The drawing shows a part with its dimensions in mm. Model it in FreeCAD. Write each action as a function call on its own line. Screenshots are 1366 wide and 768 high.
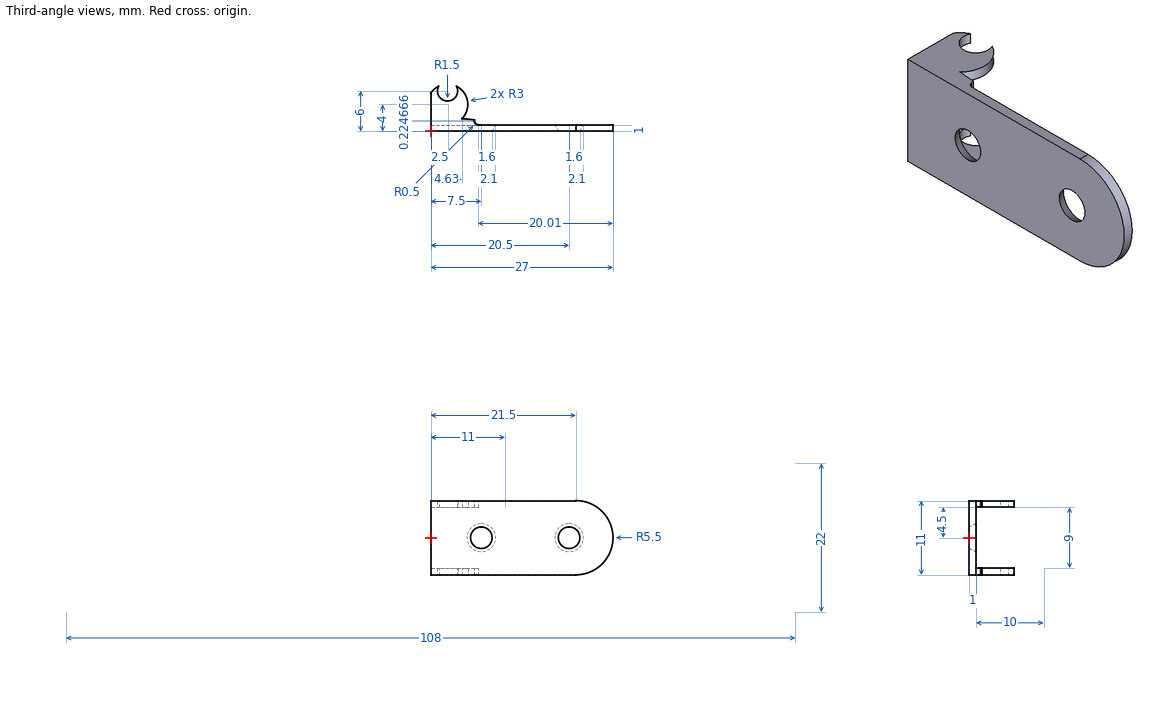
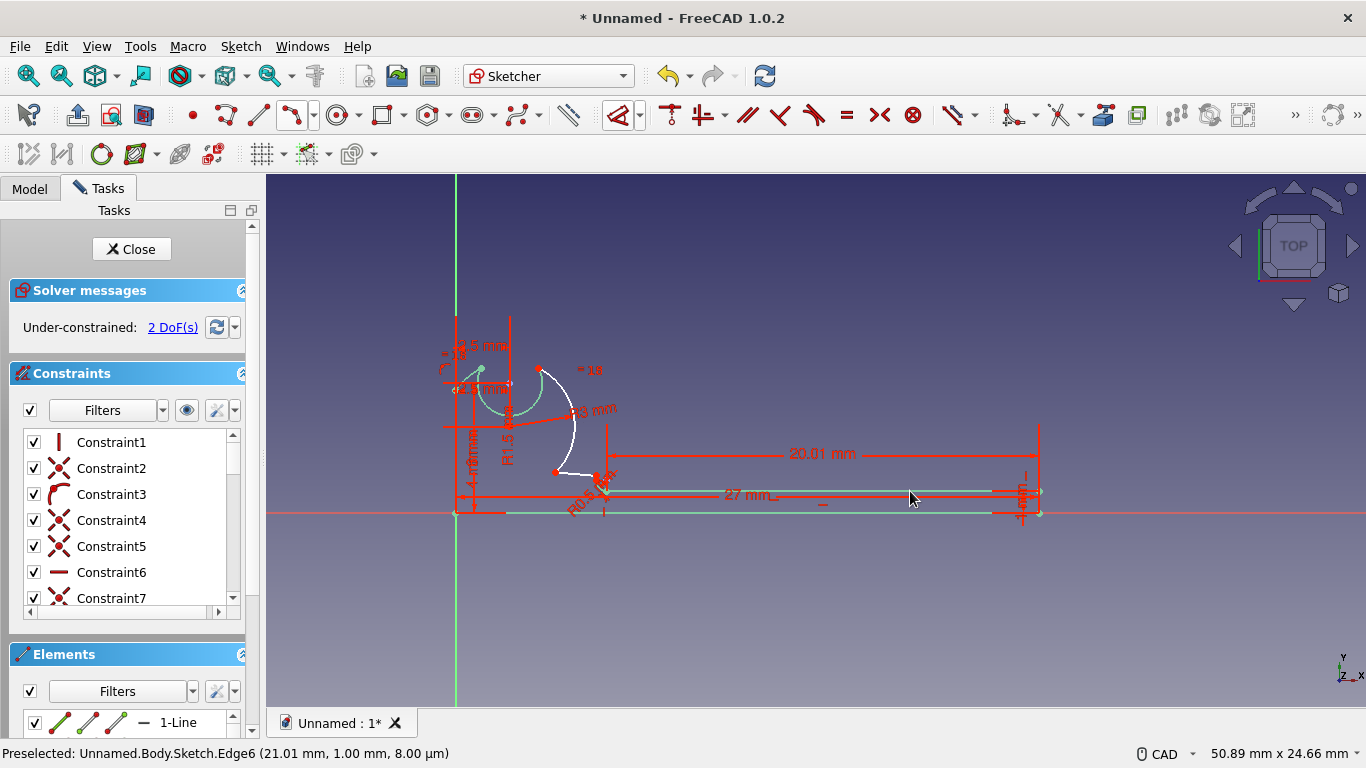
click(556, 472)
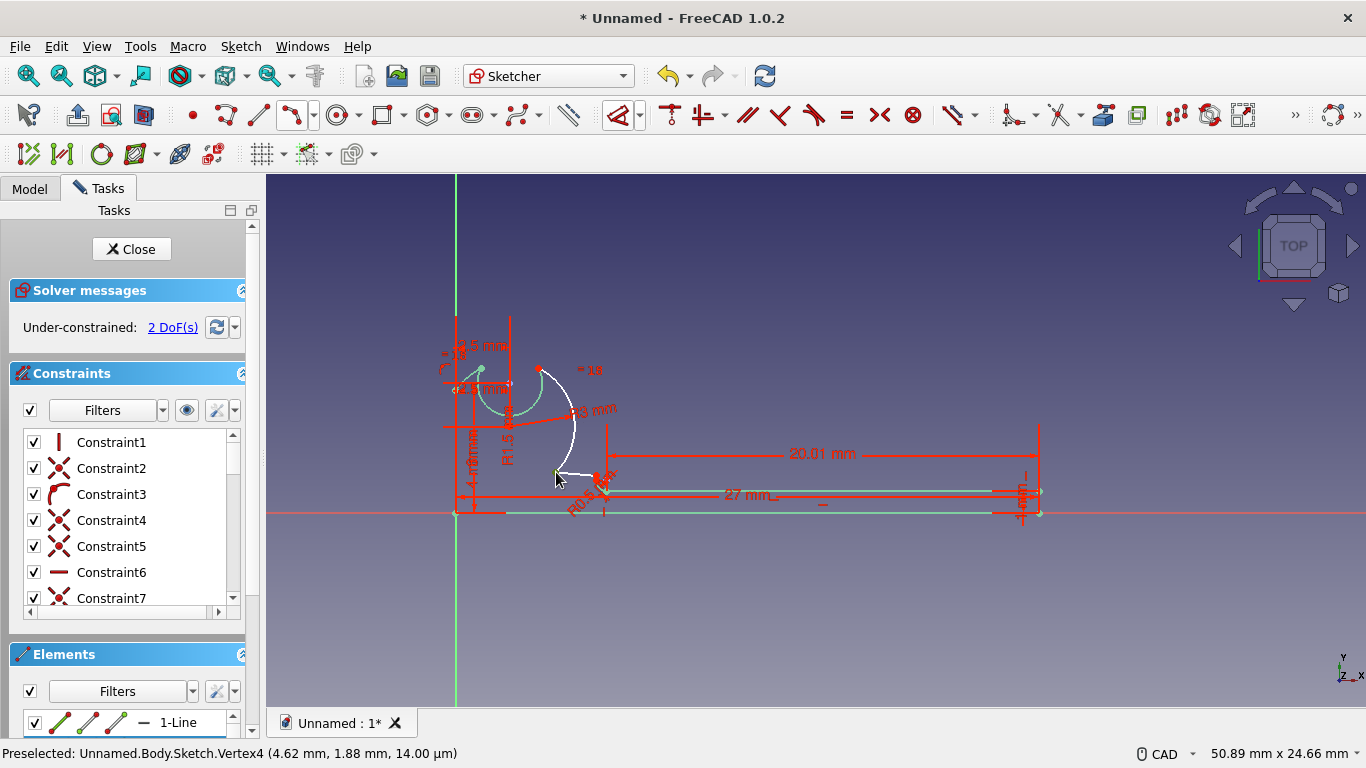
key(l)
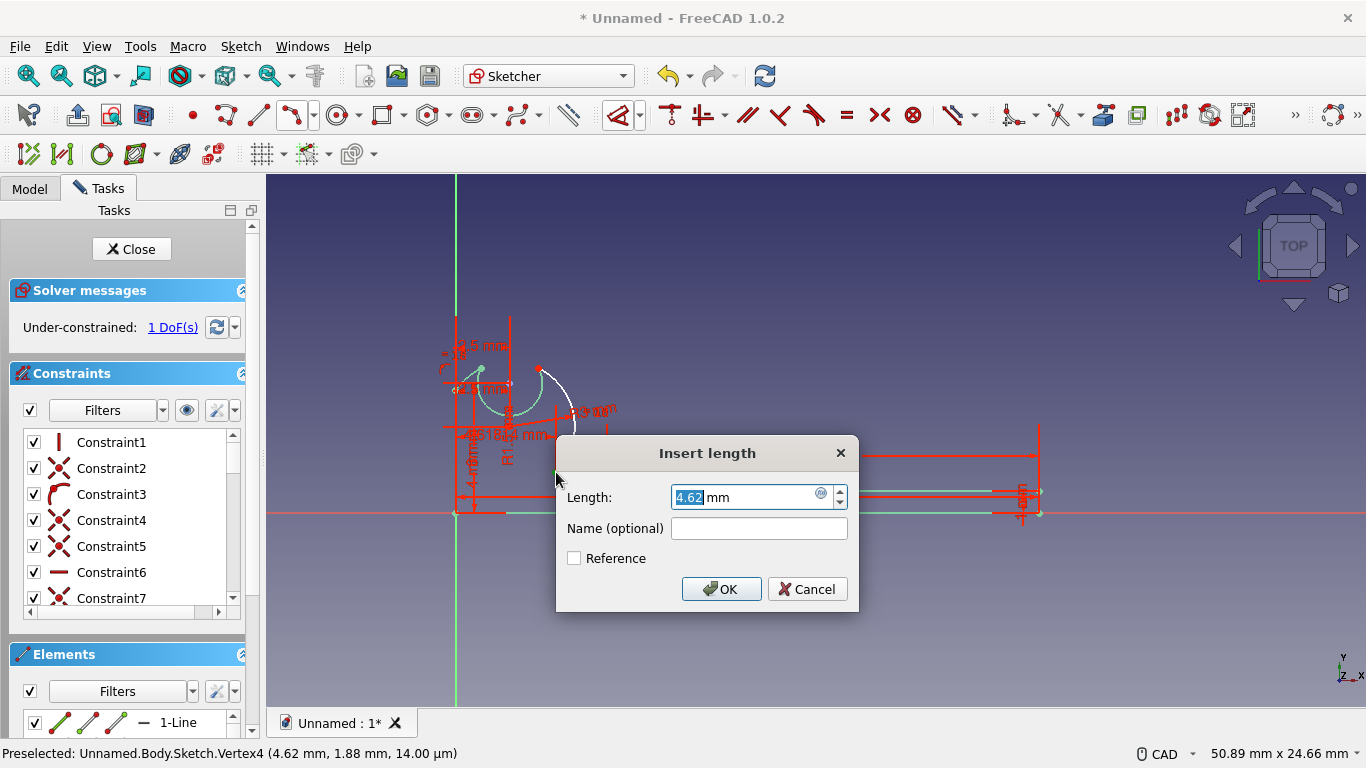
text(4.63)
key(Return)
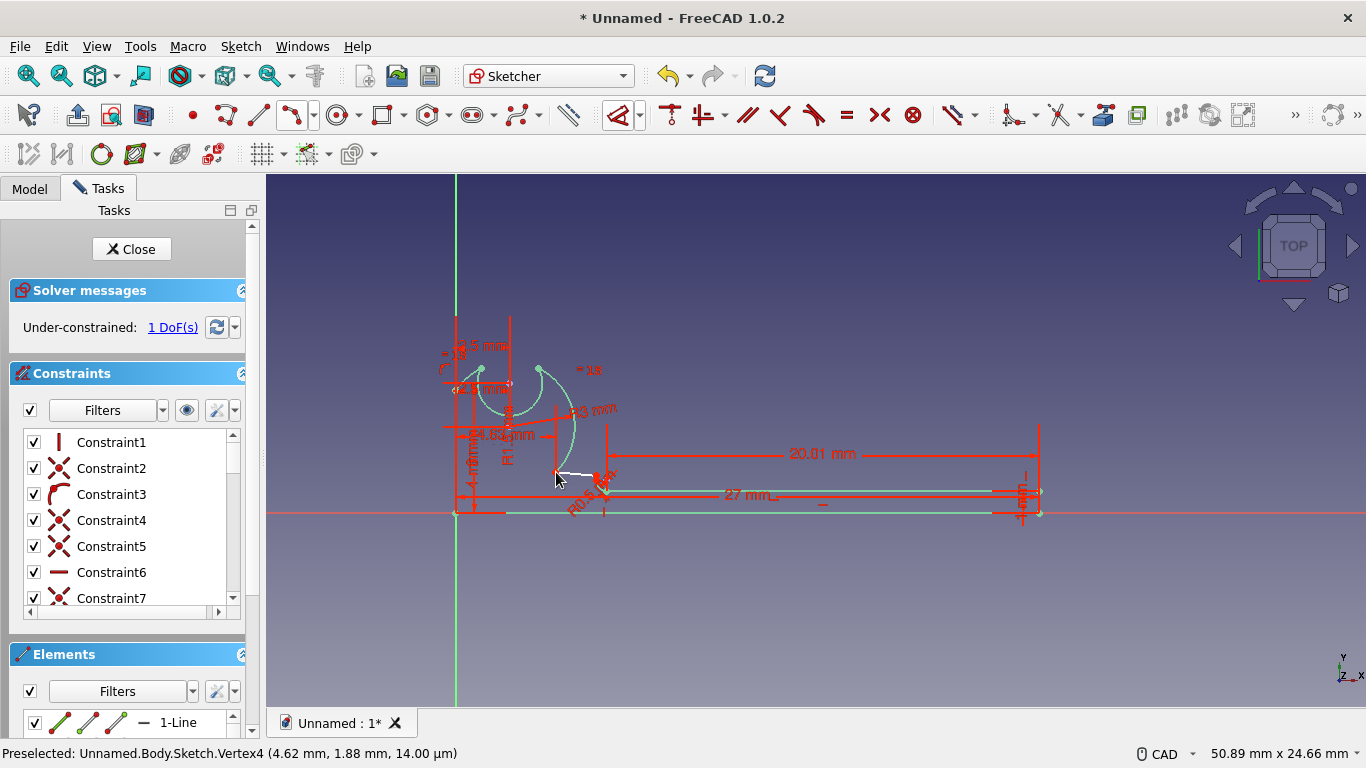
scroll(596, 478, up, 11)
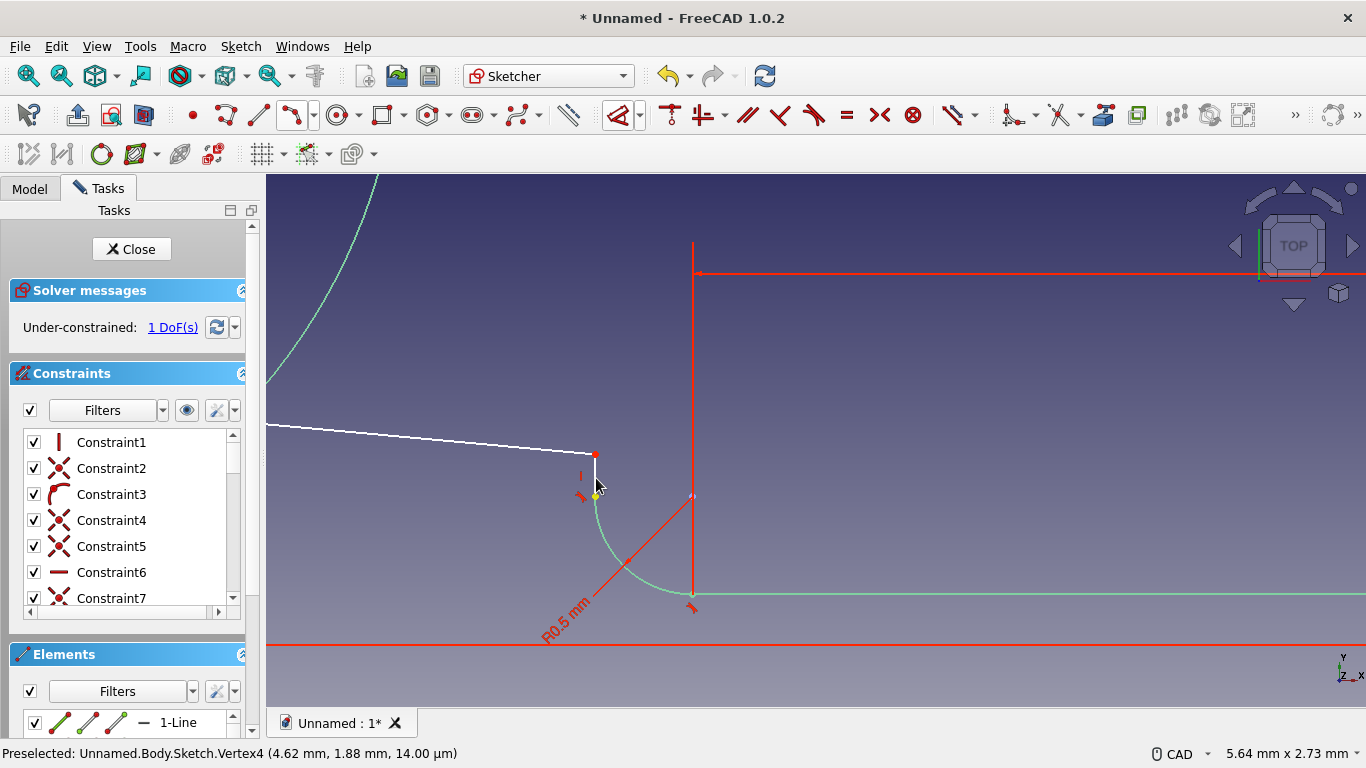
click(595, 476)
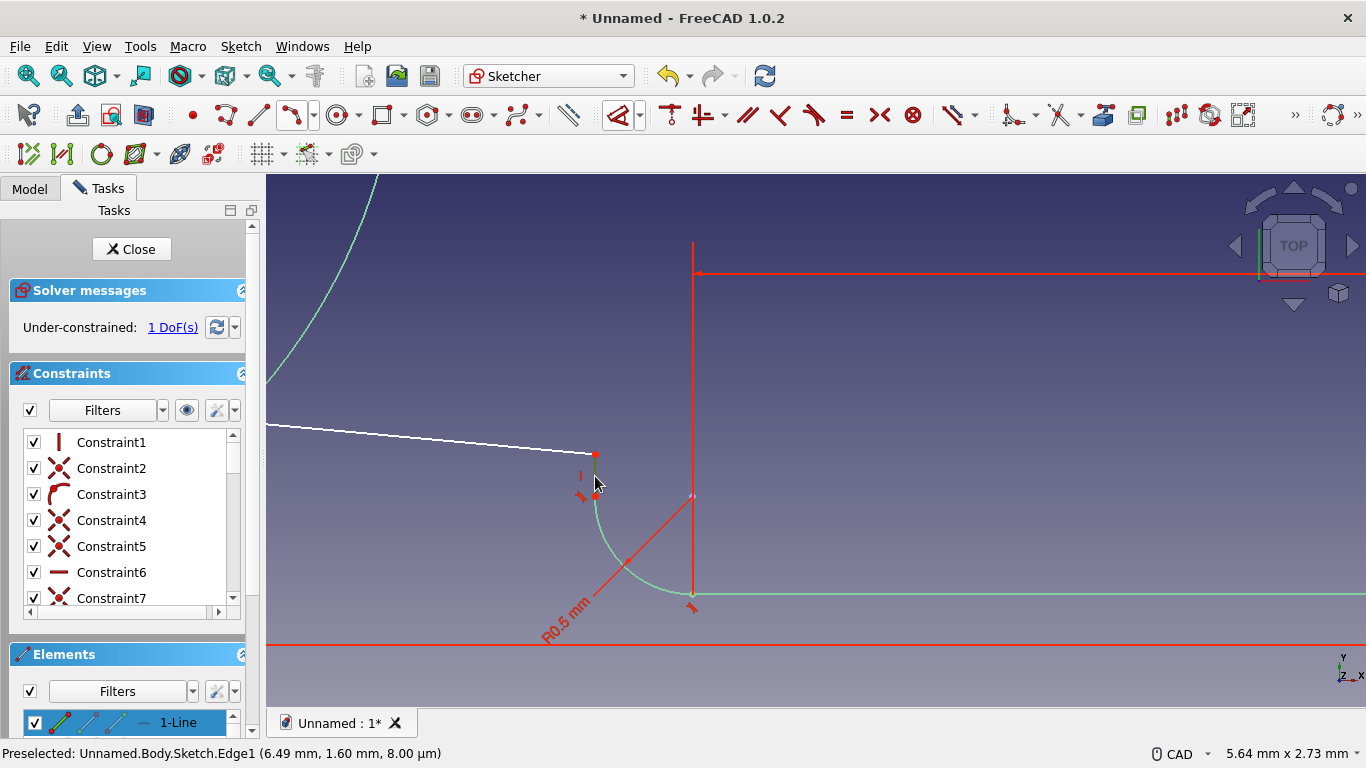
key(i)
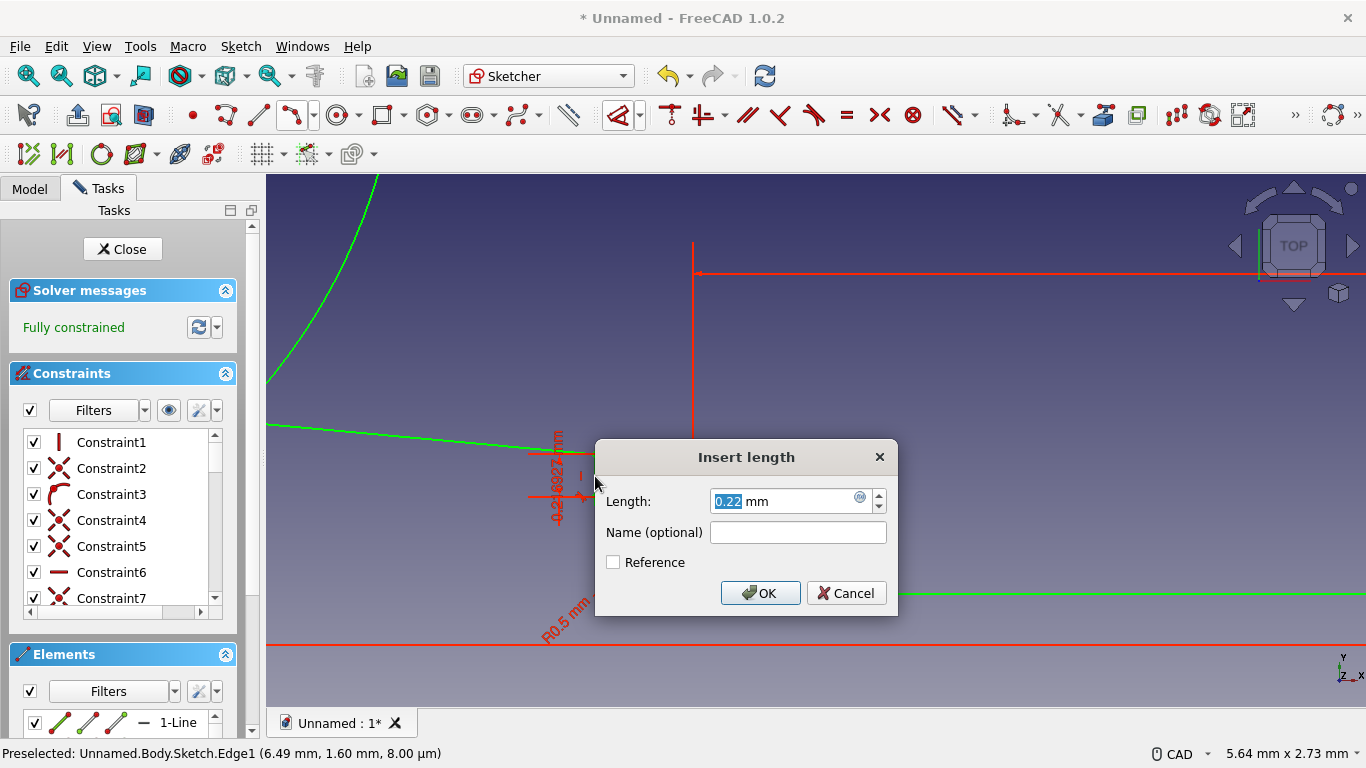
text(0.224666)
key(Return)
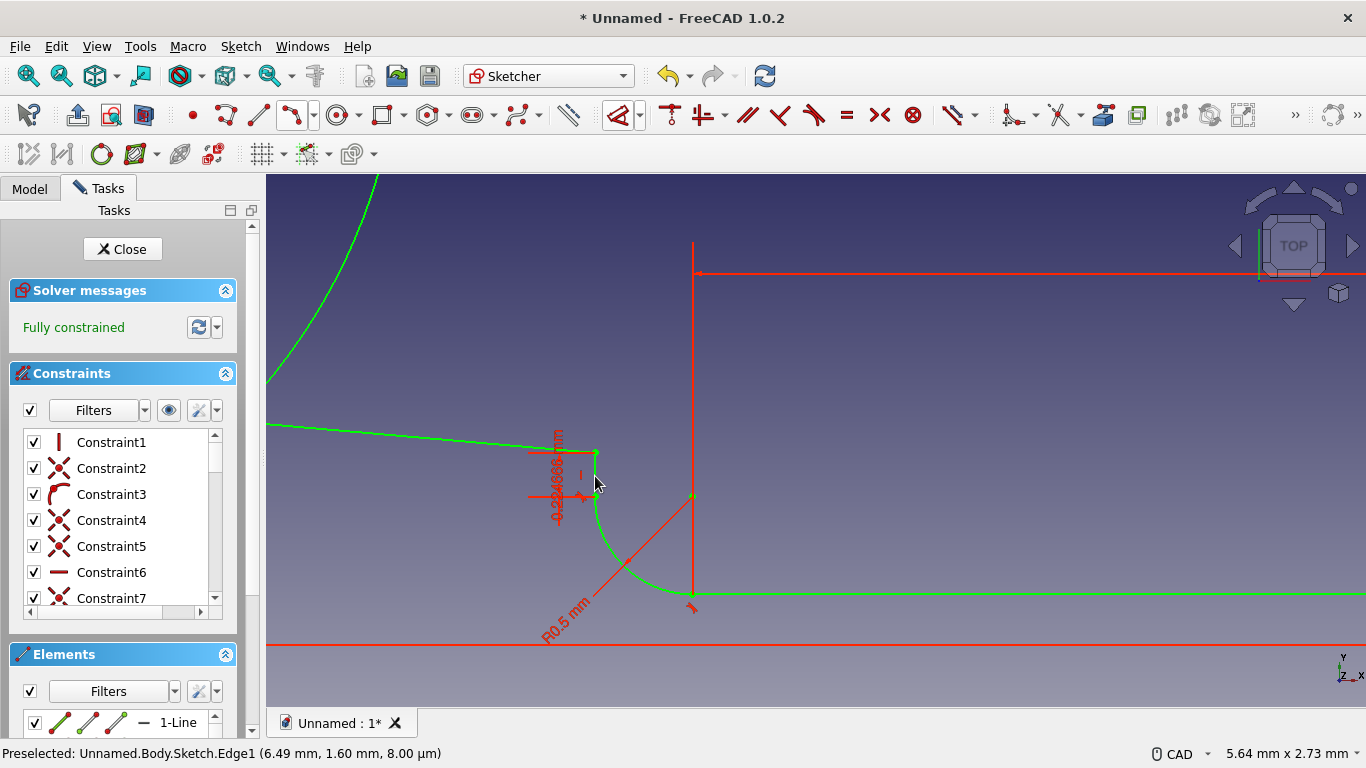
click(123, 249)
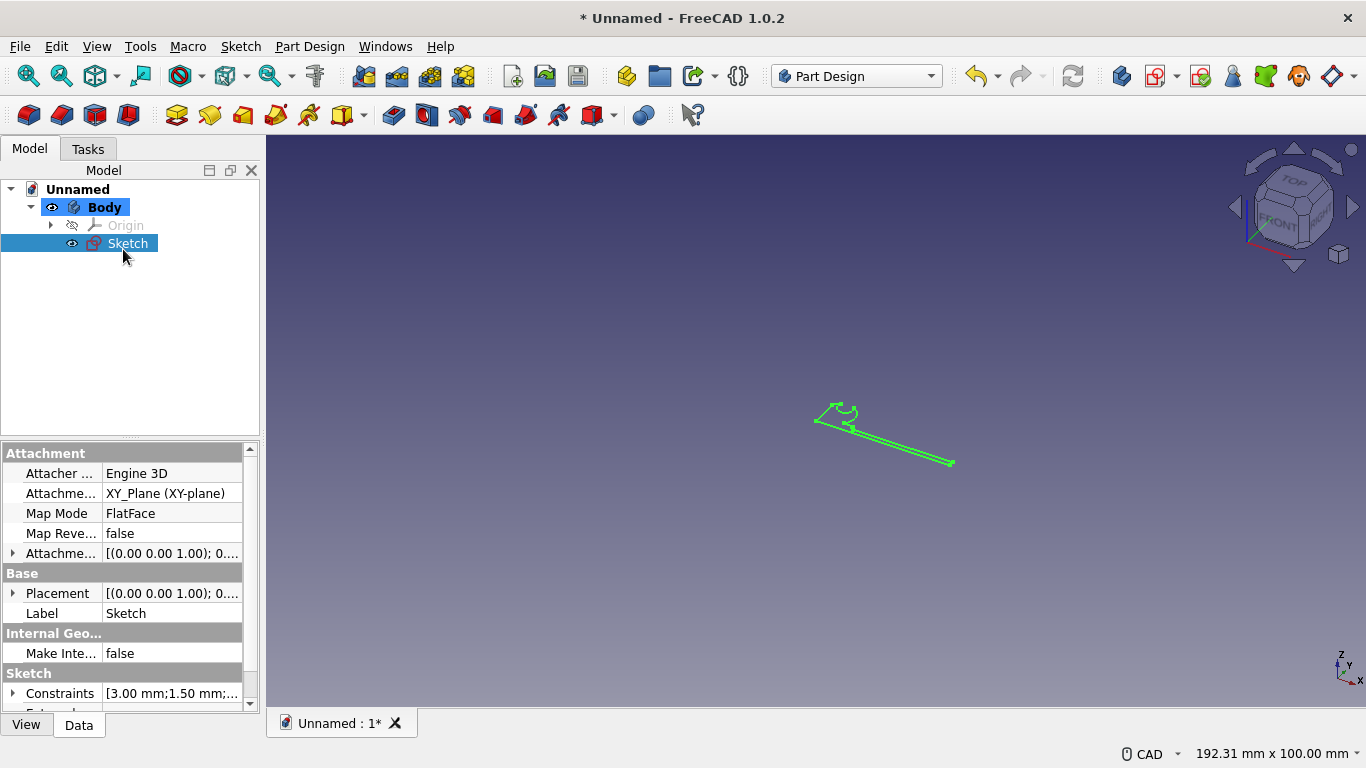
click(177, 116)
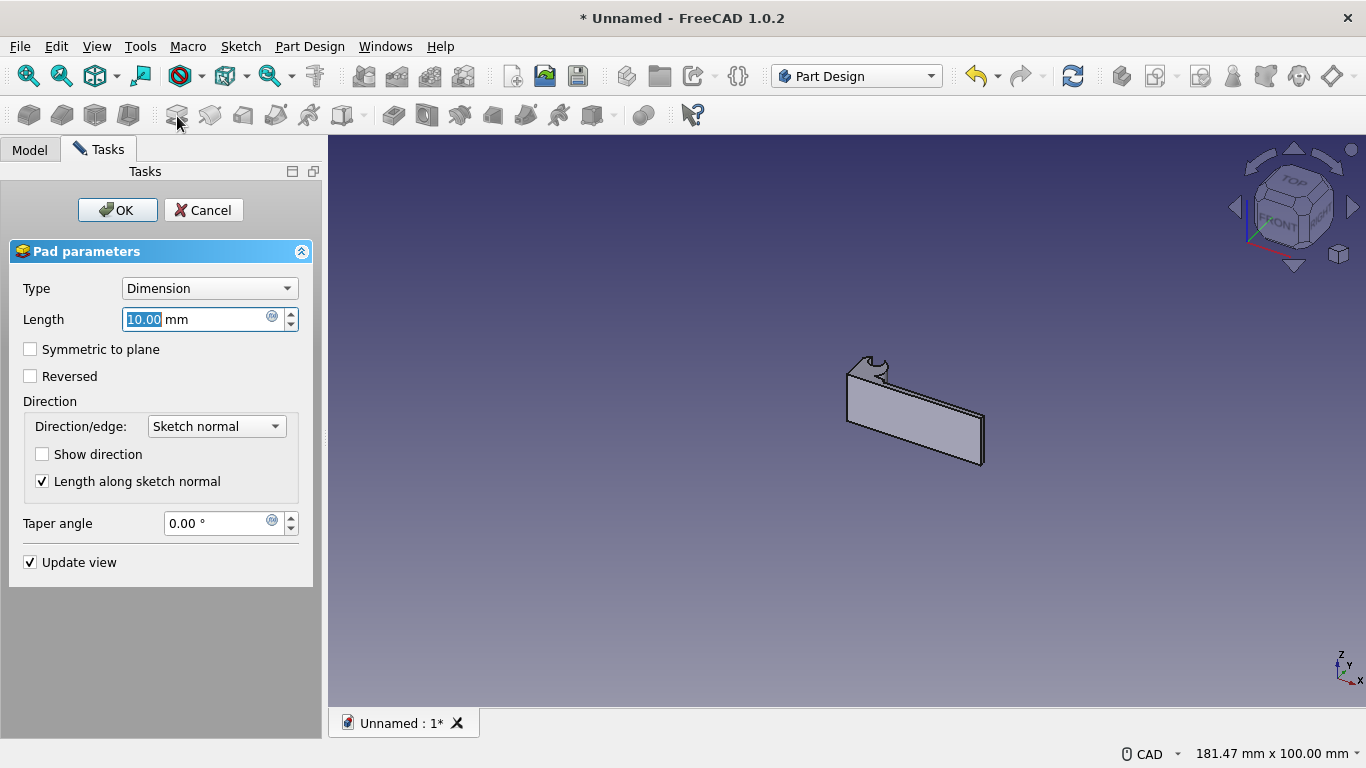
text(11)
key(Tab)